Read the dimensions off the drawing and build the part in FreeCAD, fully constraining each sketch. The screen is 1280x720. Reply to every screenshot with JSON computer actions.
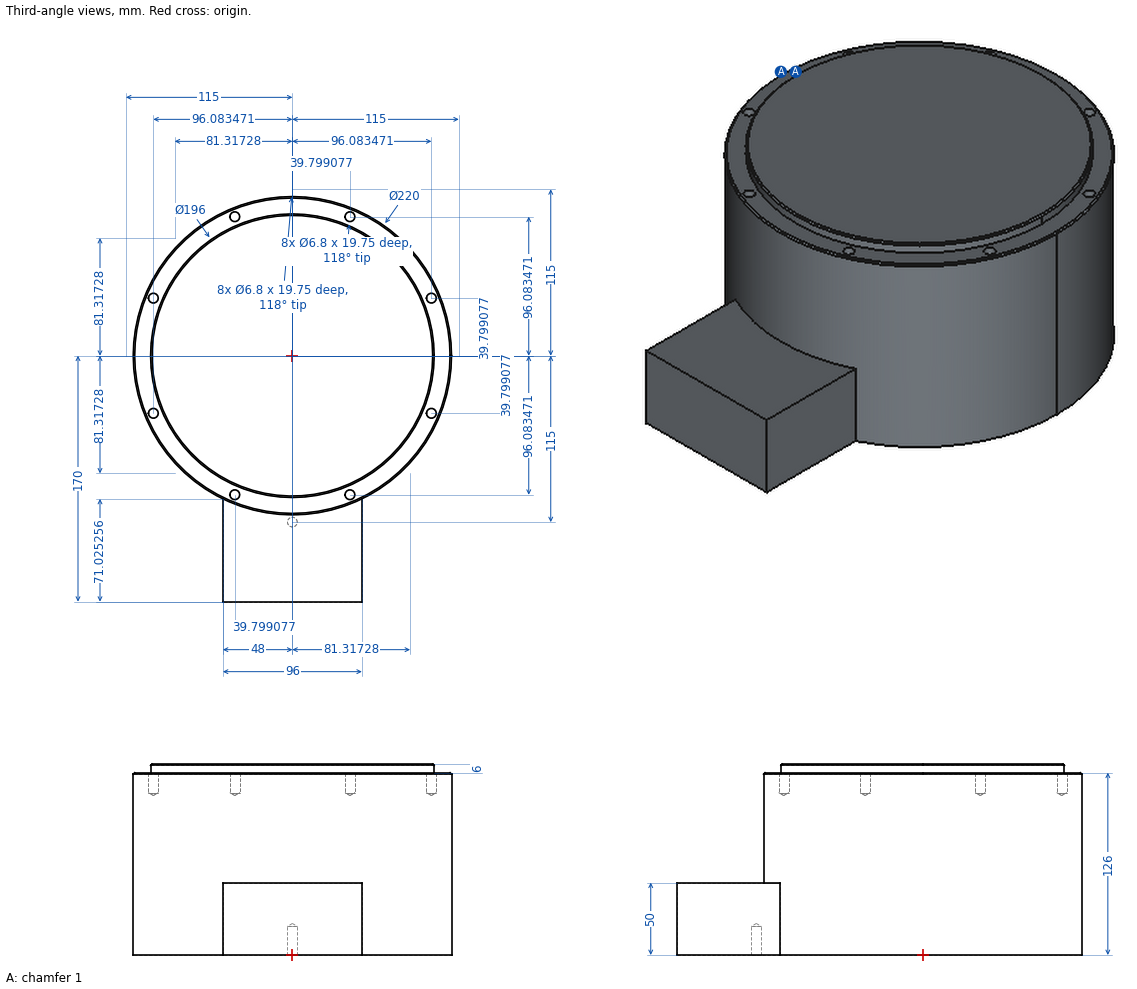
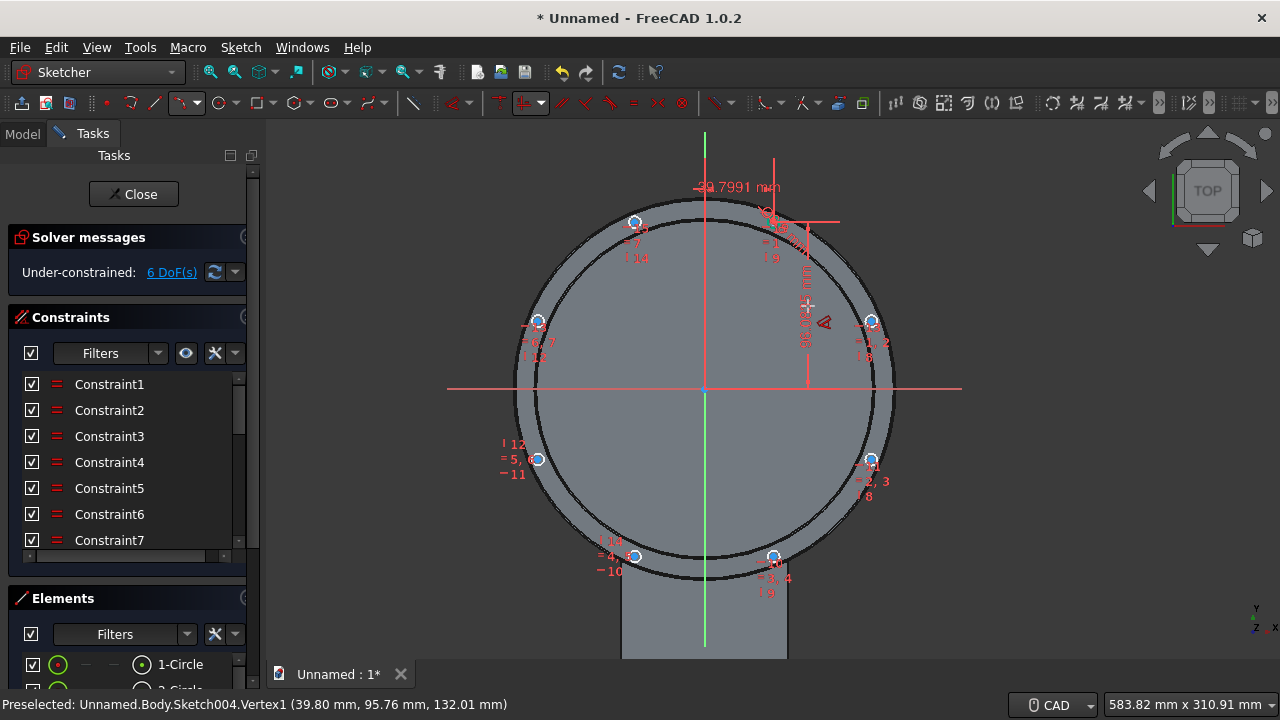
{"action": "left_click", "coordinate": [871, 321]}
{"action": "left_click", "coordinate": [730, 287]}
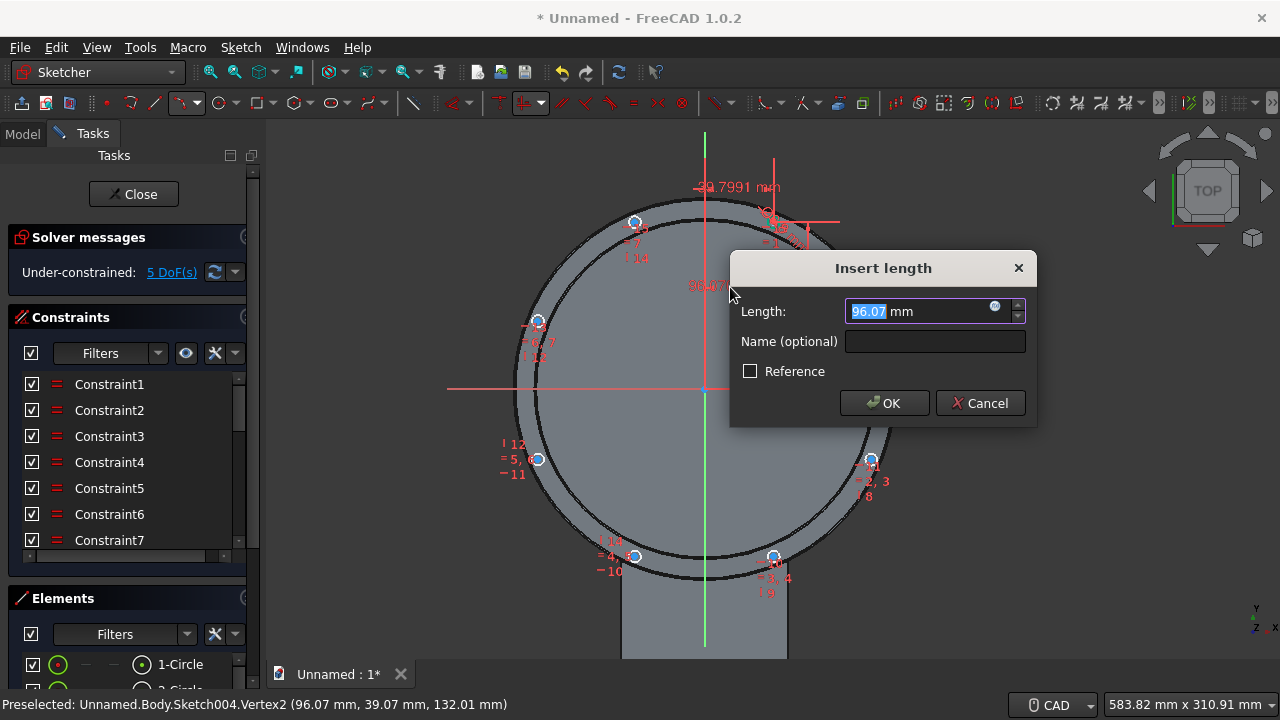
{"action": "type", "text": "96.083471"}
{"action": "key", "text": "Return"}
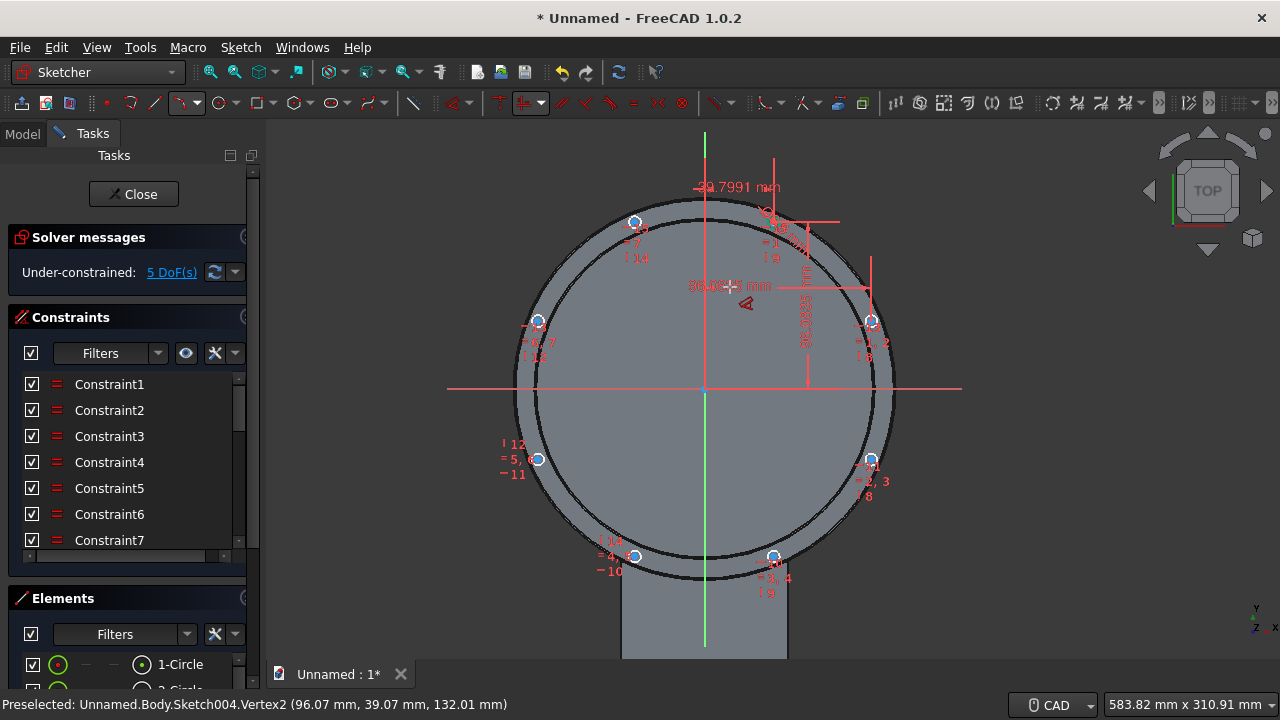
{"action": "left_click", "coordinate": [871, 321]}
{"action": "left_click", "coordinate": [905, 355]}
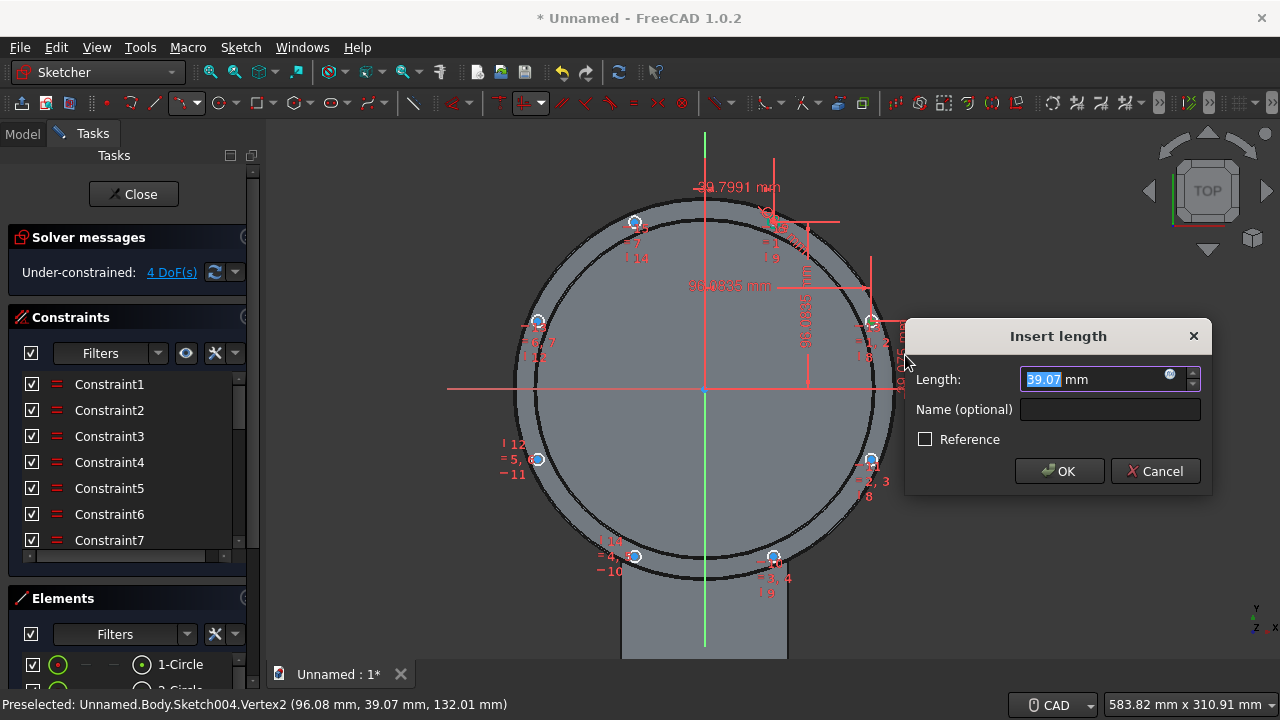
{"action": "type", "text": "39.799077"}
{"action": "key", "text": "Return"}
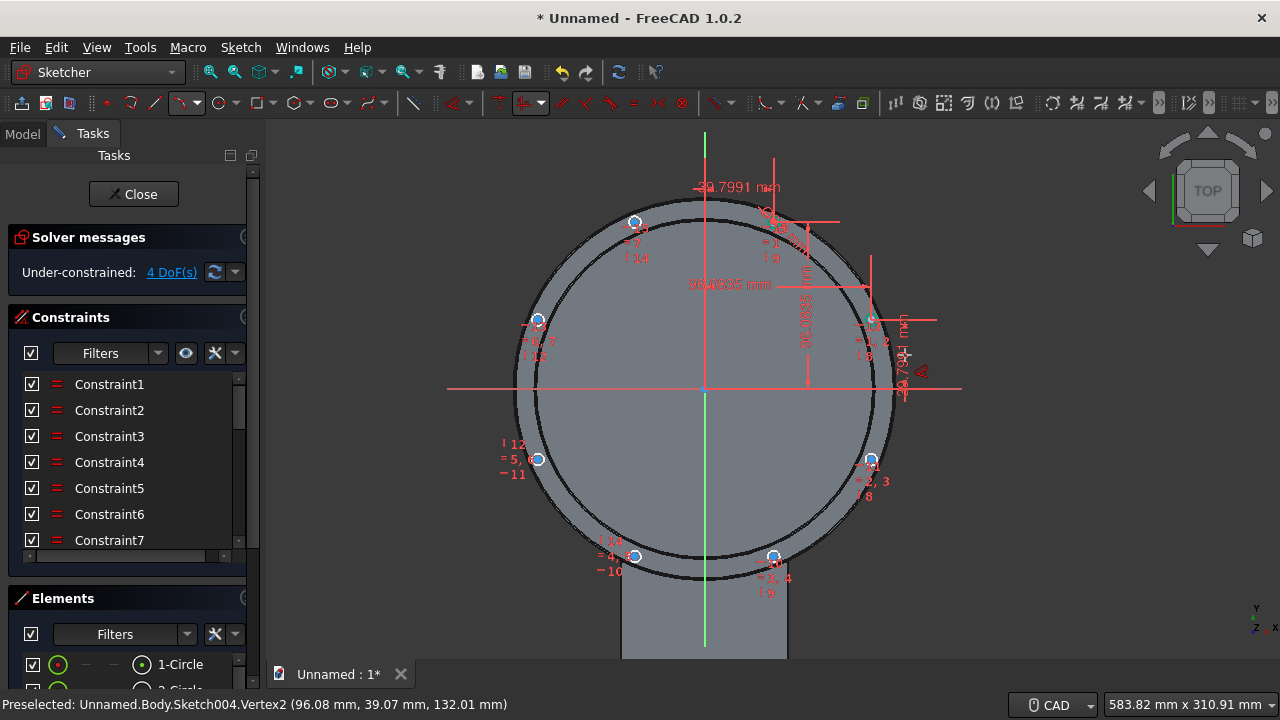
{"action": "left_click", "coordinate": [871, 460]}
{"action": "left_click", "coordinate": [905, 424]}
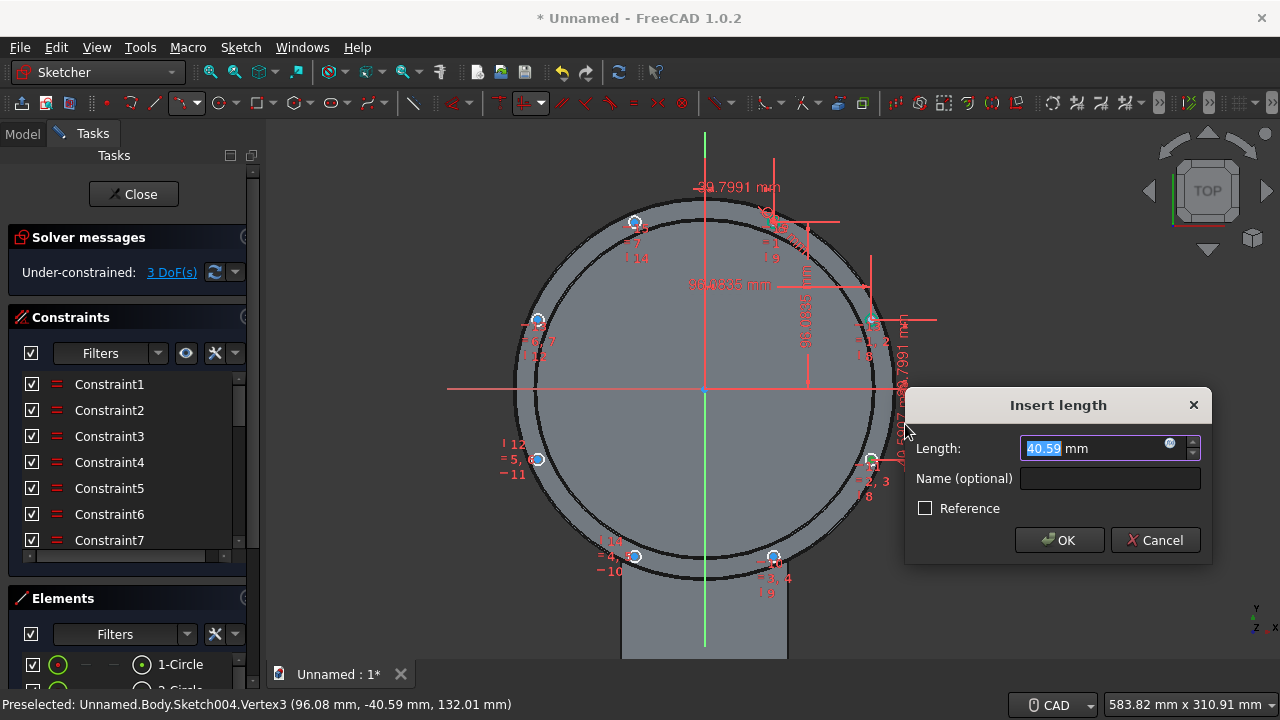
{"action": "type", "text": "39.799077"}
{"action": "key", "text": "Return"}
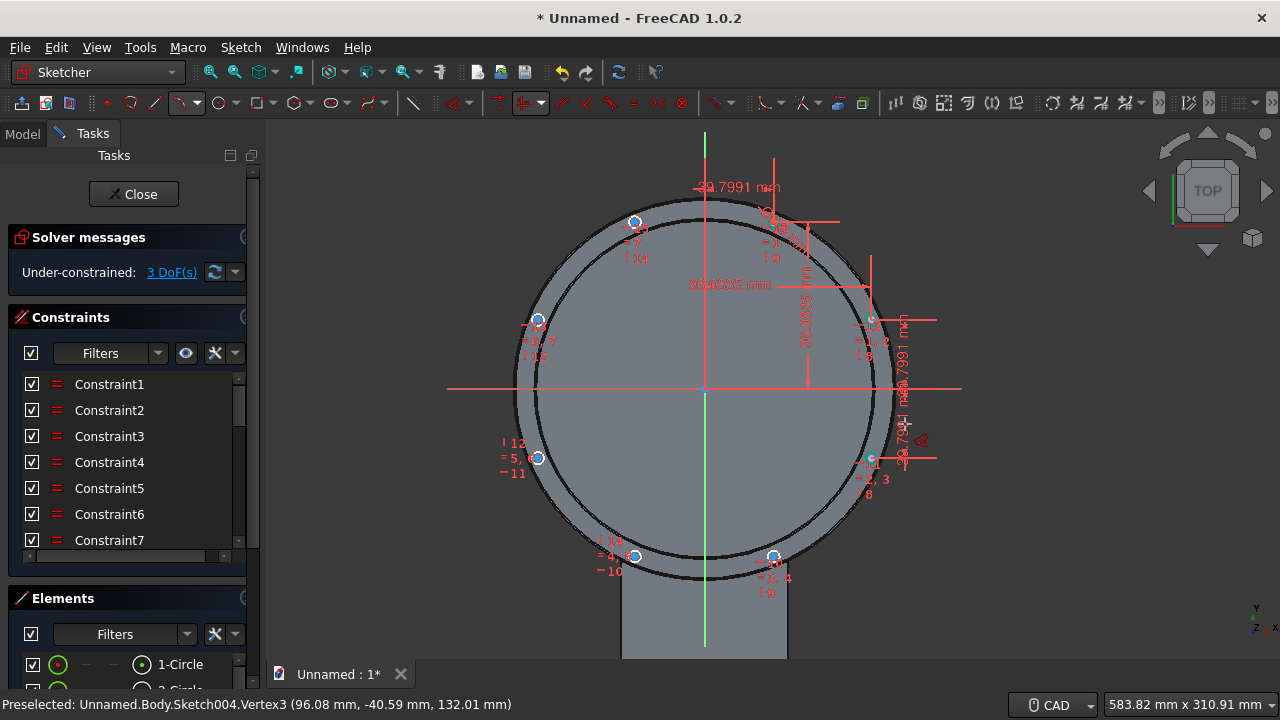
{"action": "left_click", "coordinate": [774, 557]}
{"action": "left_click", "coordinate": [808, 473]}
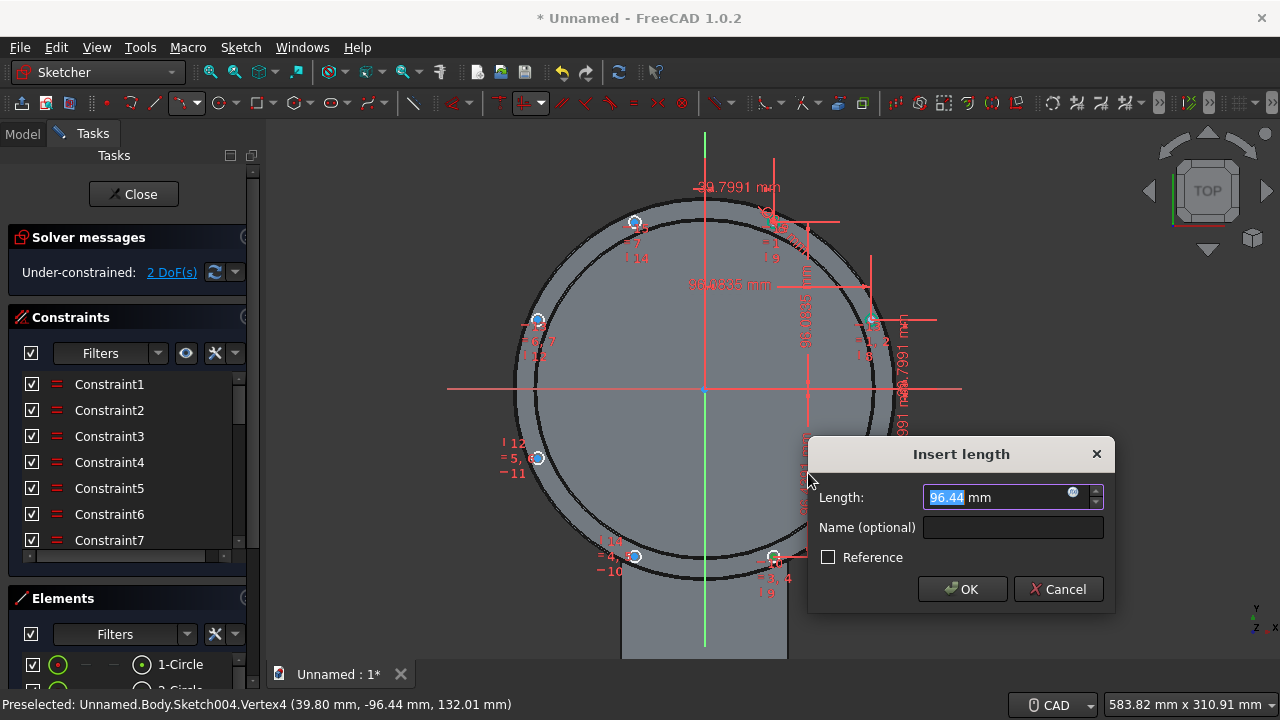
{"action": "type", "text": "96.083471"}
{"action": "key", "text": "Return"}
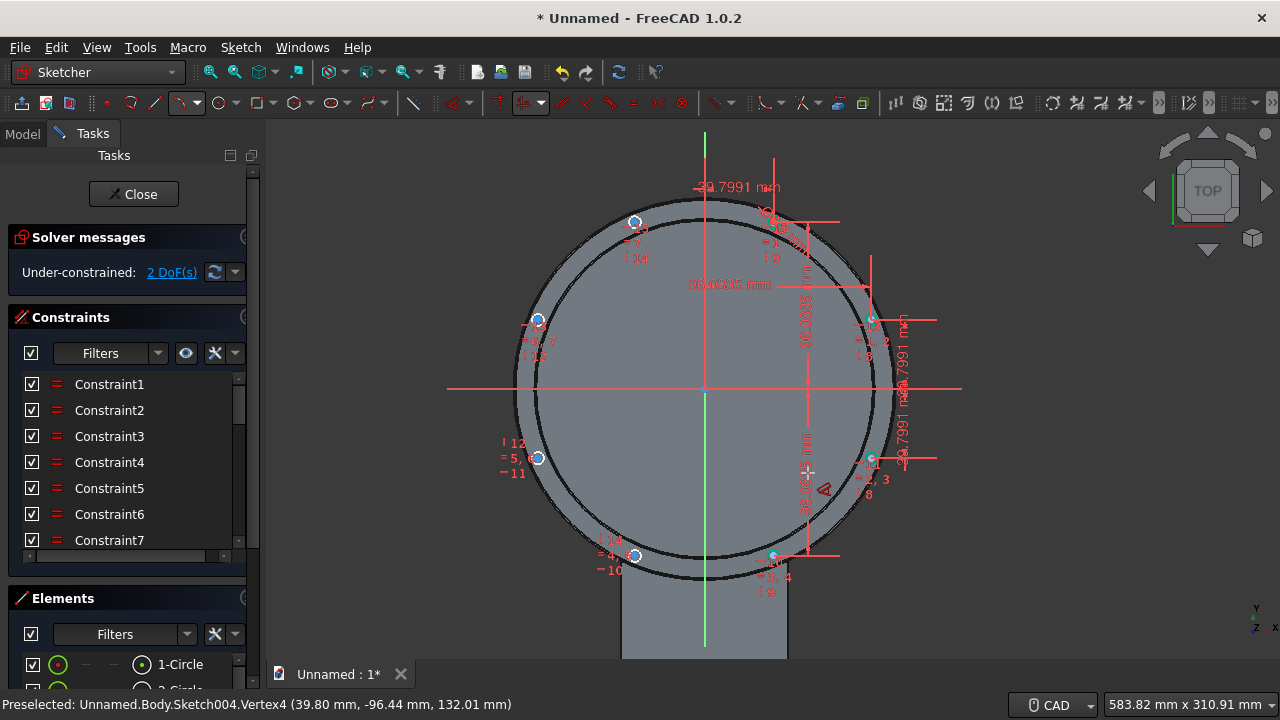
{"action": "left_click", "coordinate": [635, 556]}
{"action": "left_click", "coordinate": [670, 590]}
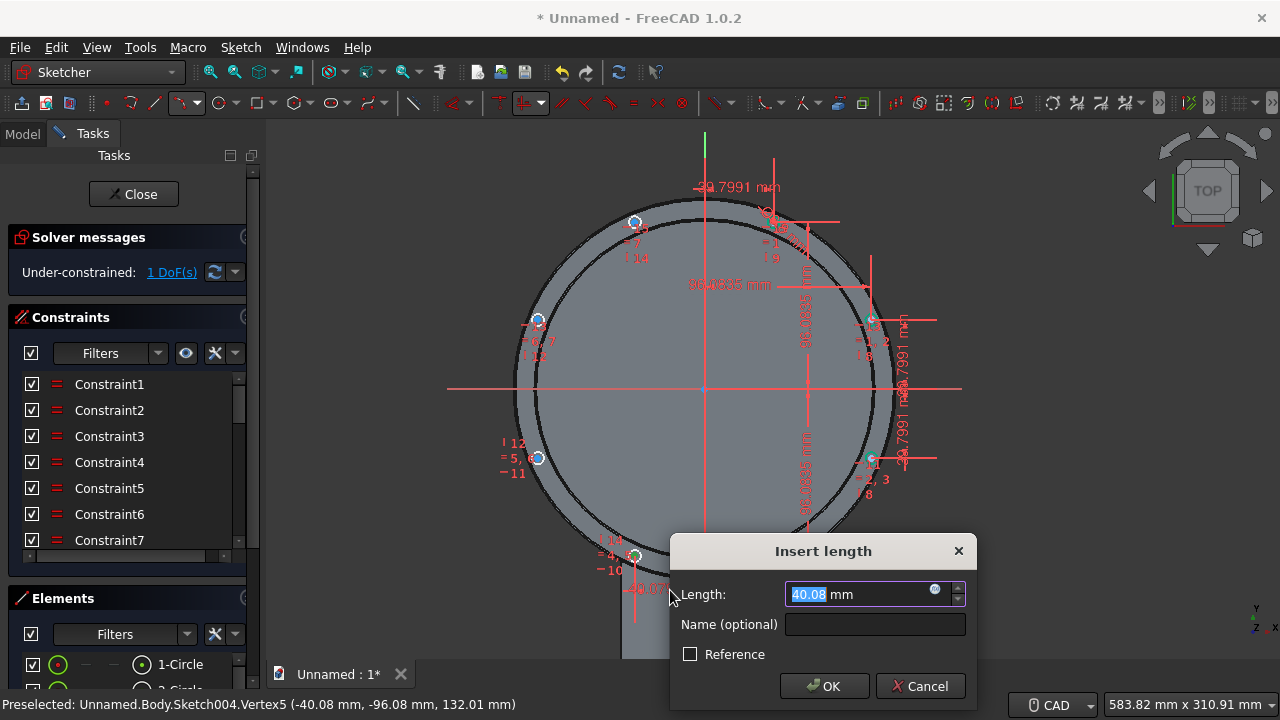
{"action": "type", "text": "39.799077"}
{"action": "key", "text": "Return"}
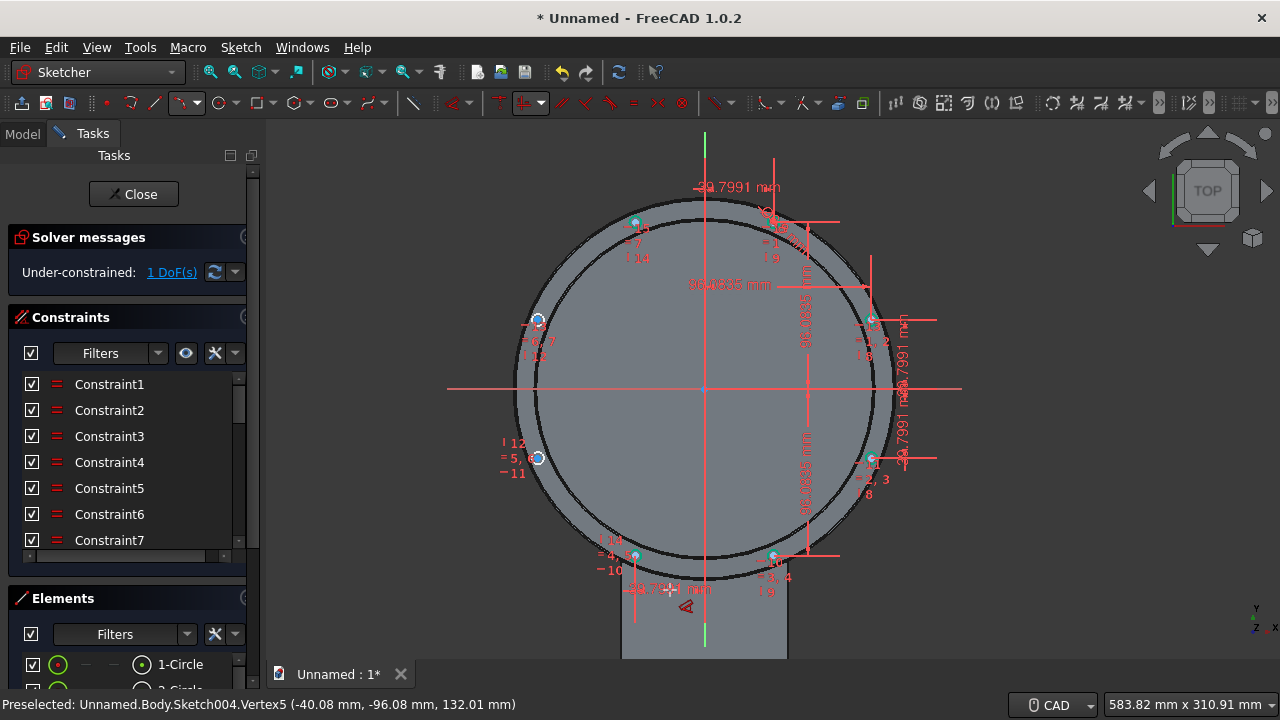
{"action": "left_click", "coordinate": [538, 458]}
{"action": "left_click", "coordinate": [621, 492]}